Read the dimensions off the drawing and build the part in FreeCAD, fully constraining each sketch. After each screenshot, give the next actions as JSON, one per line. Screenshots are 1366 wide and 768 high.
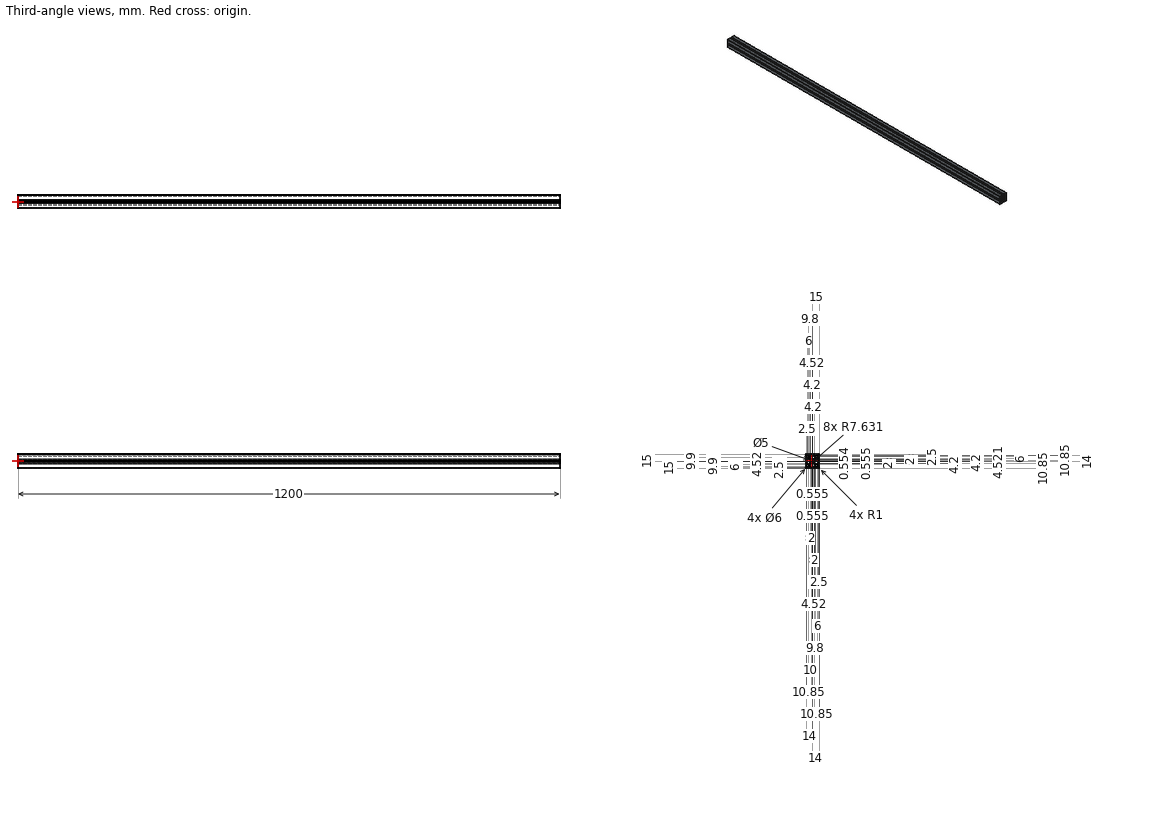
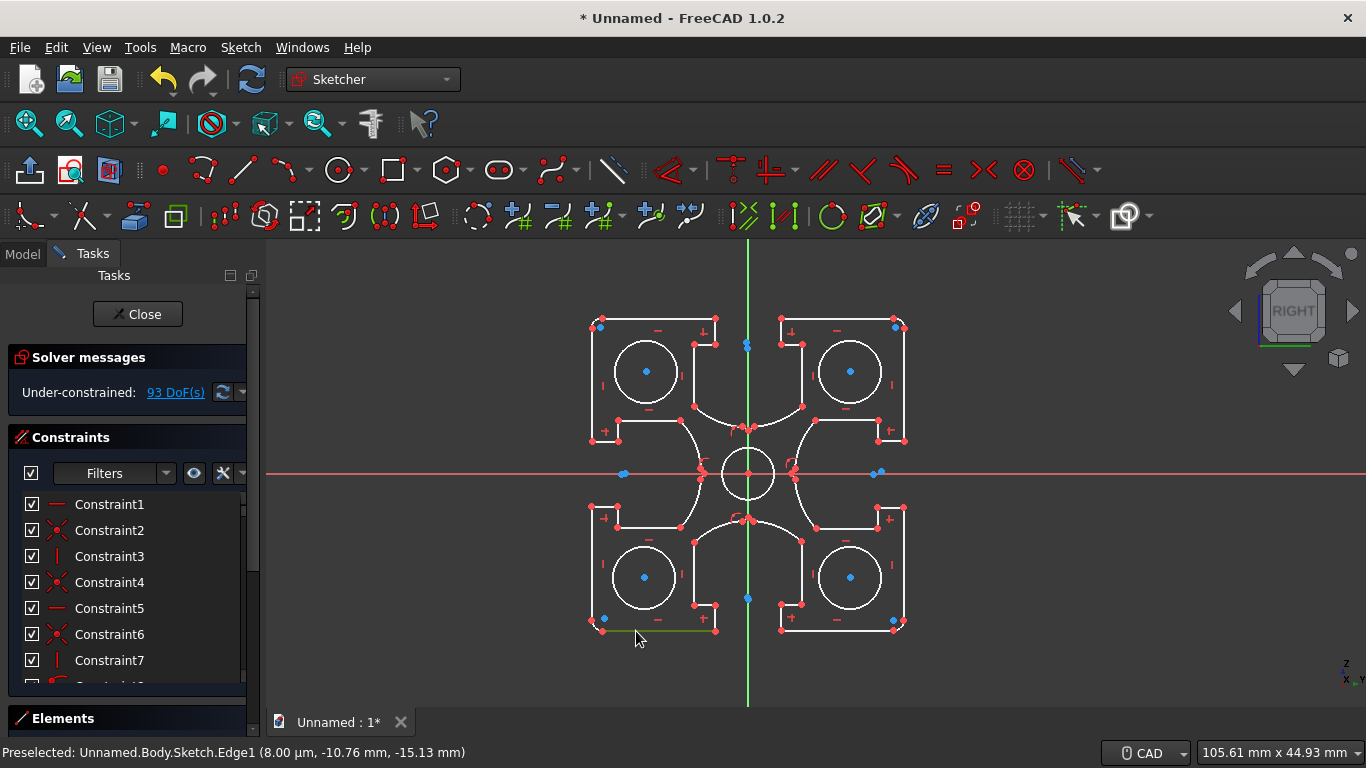
{"action": "scroll", "coordinate": [595, 628], "scroll_direction": "up", "scroll_amount": 3}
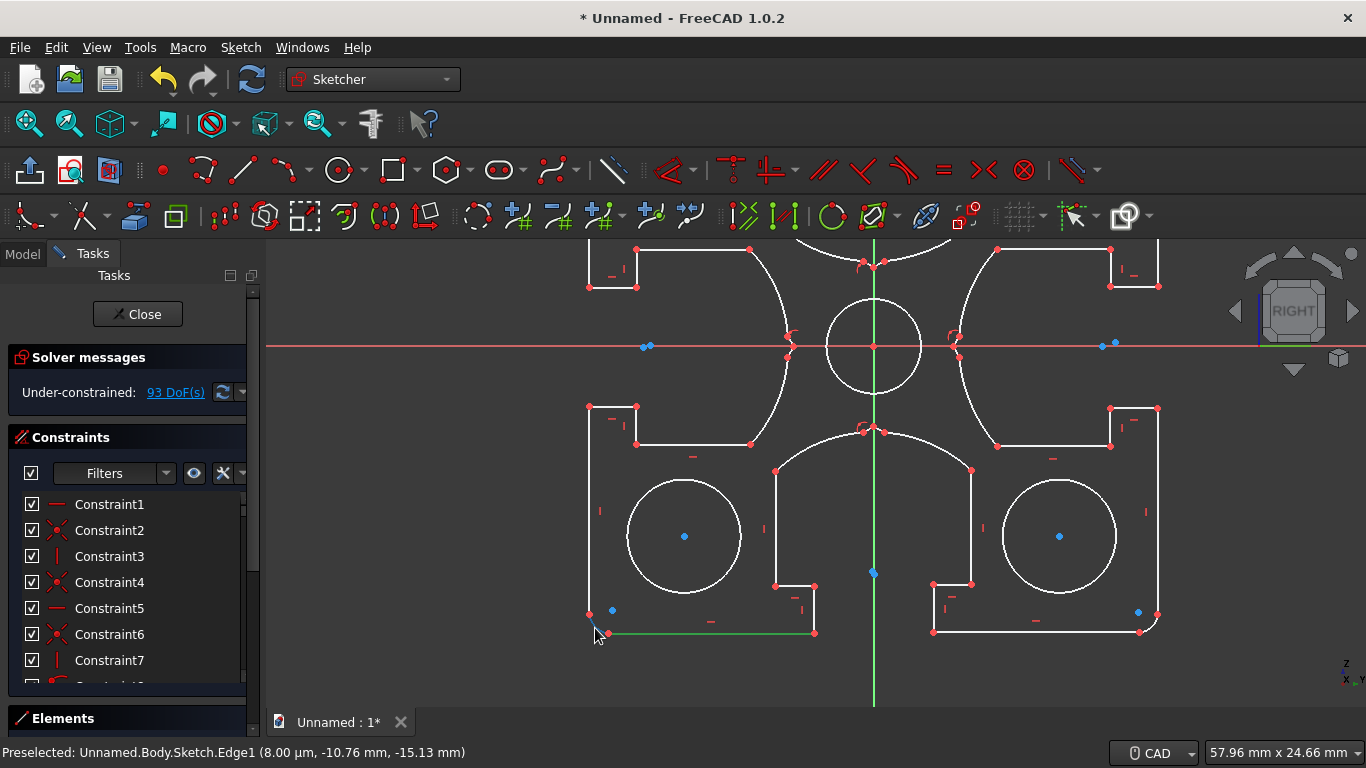
{"action": "left_click", "coordinate": [596, 627]}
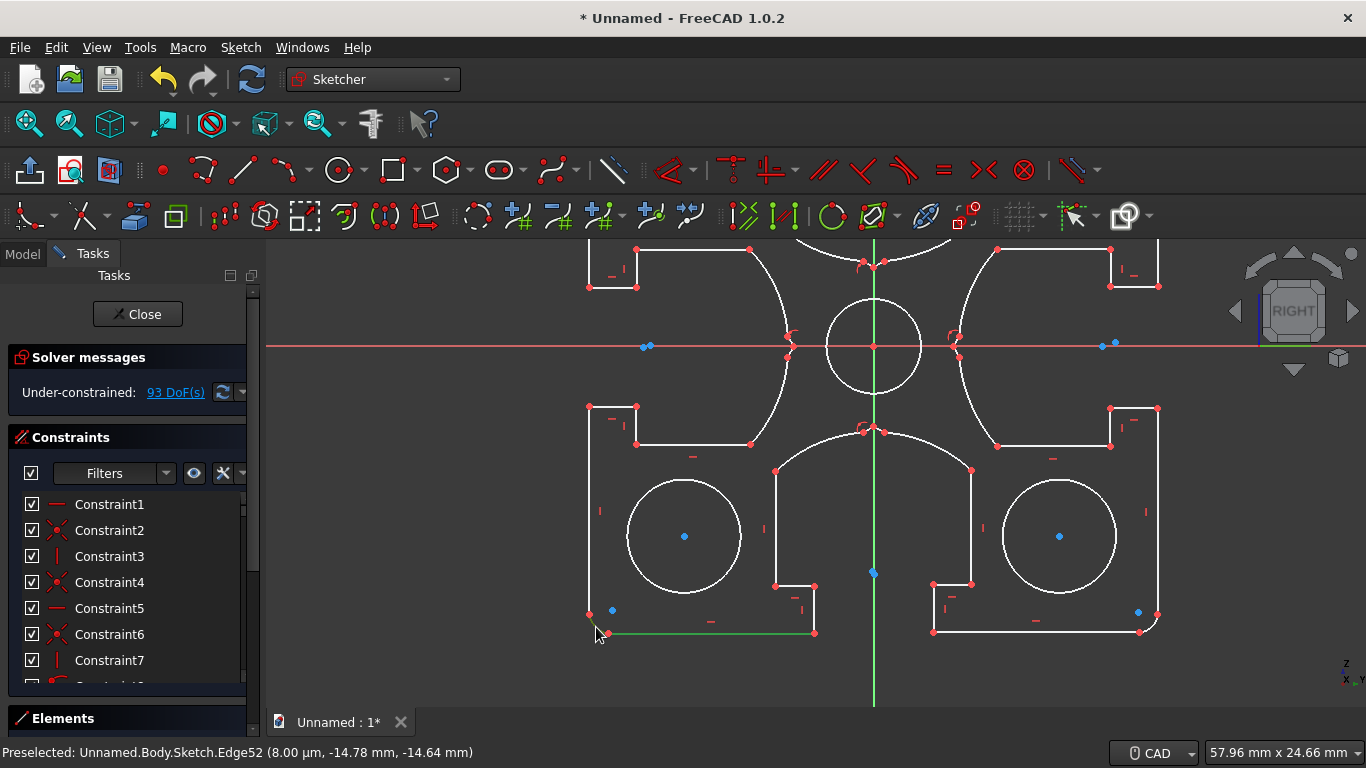
{"action": "left_click", "coordinate": [904, 170]}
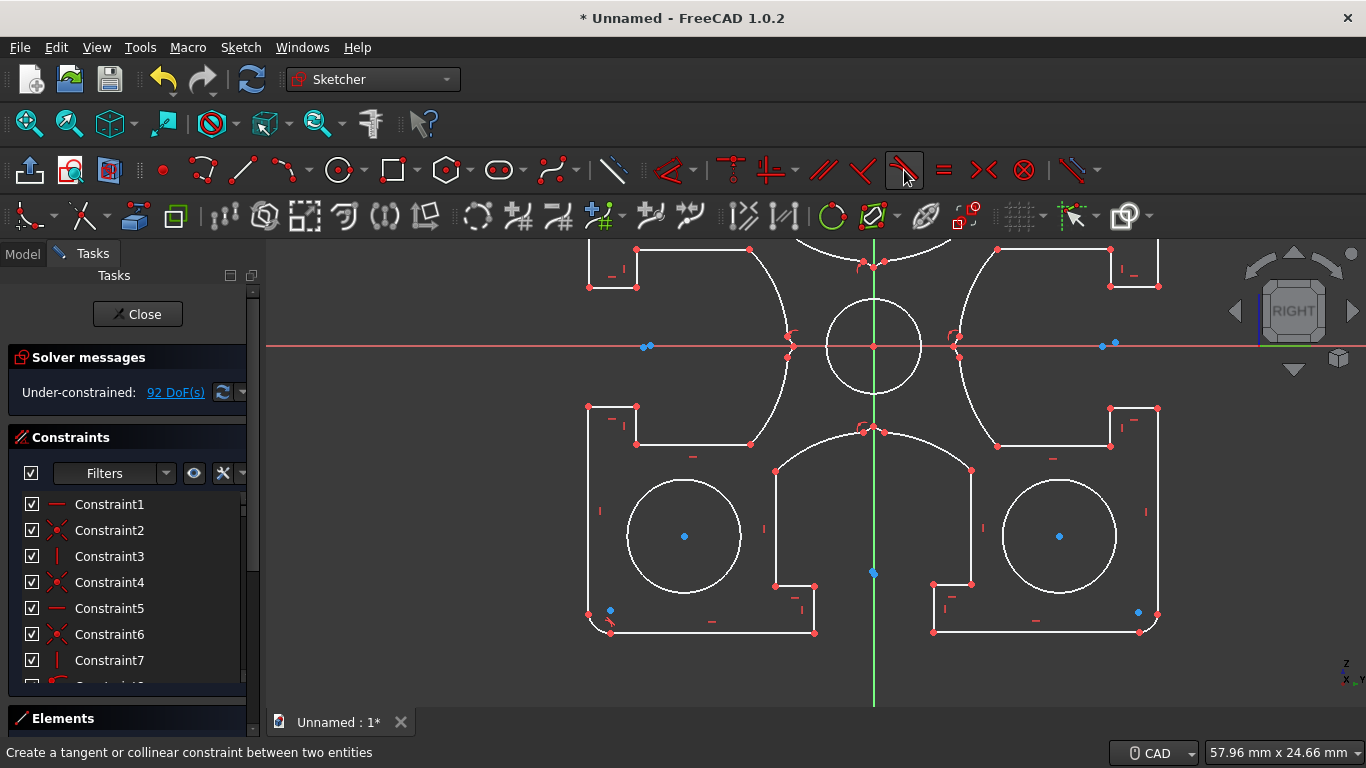
{"action": "left_click", "coordinate": [995, 632]}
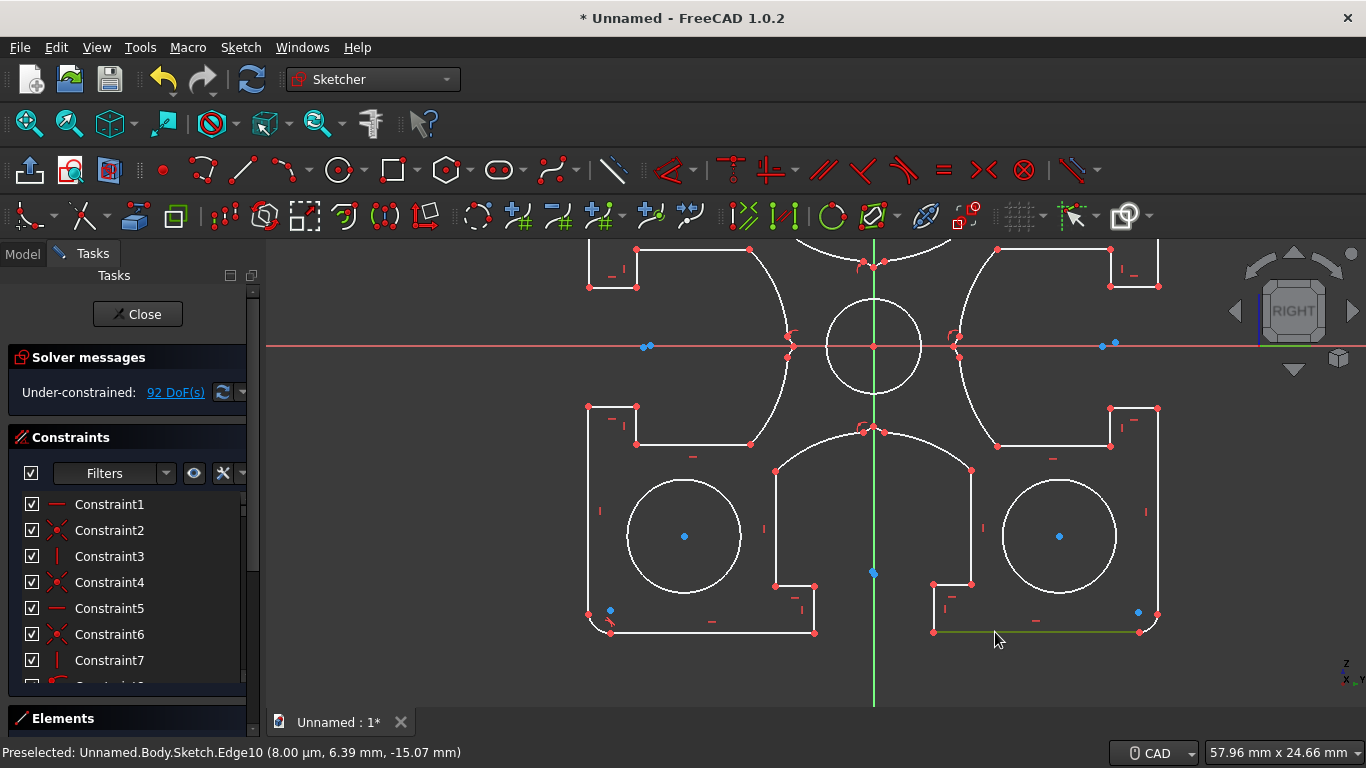
{"action": "left_click", "coordinate": [1152, 627]}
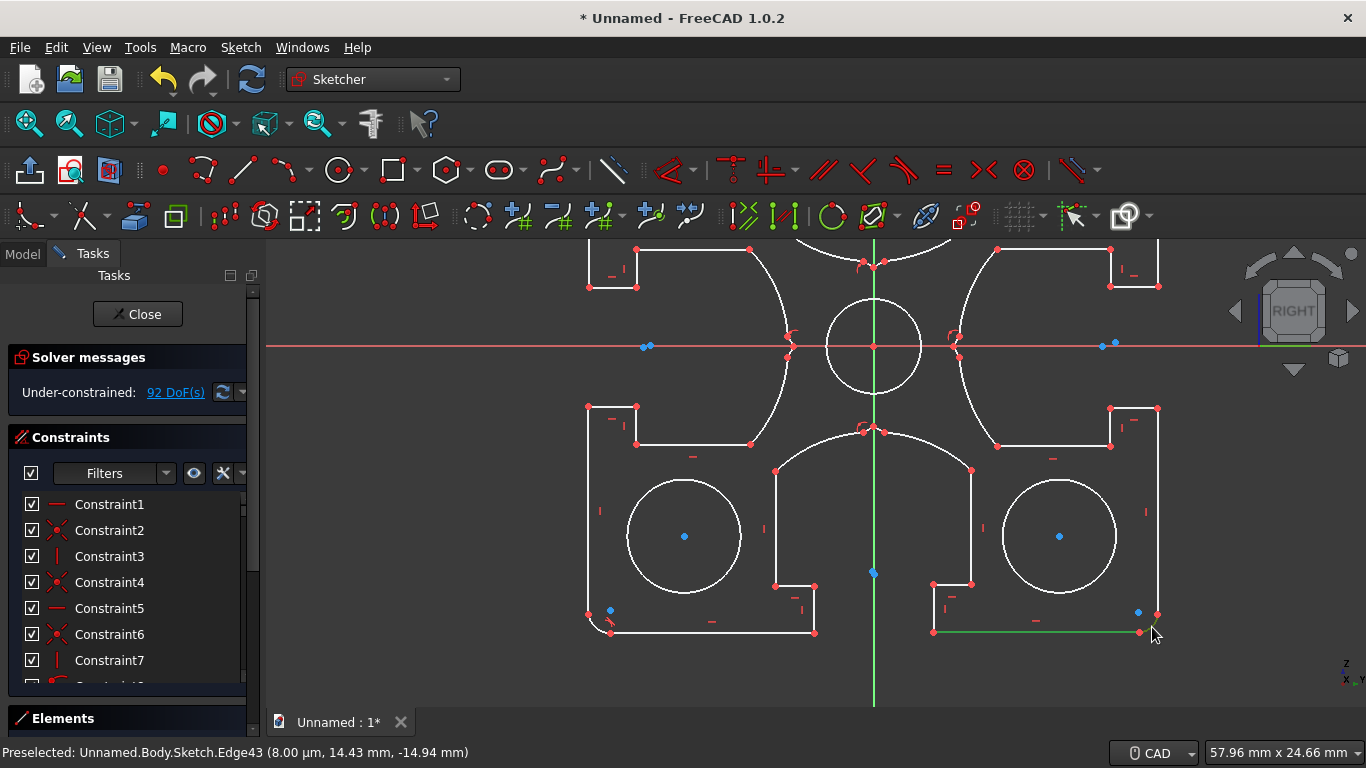
{"action": "left_click", "coordinate": [904, 170]}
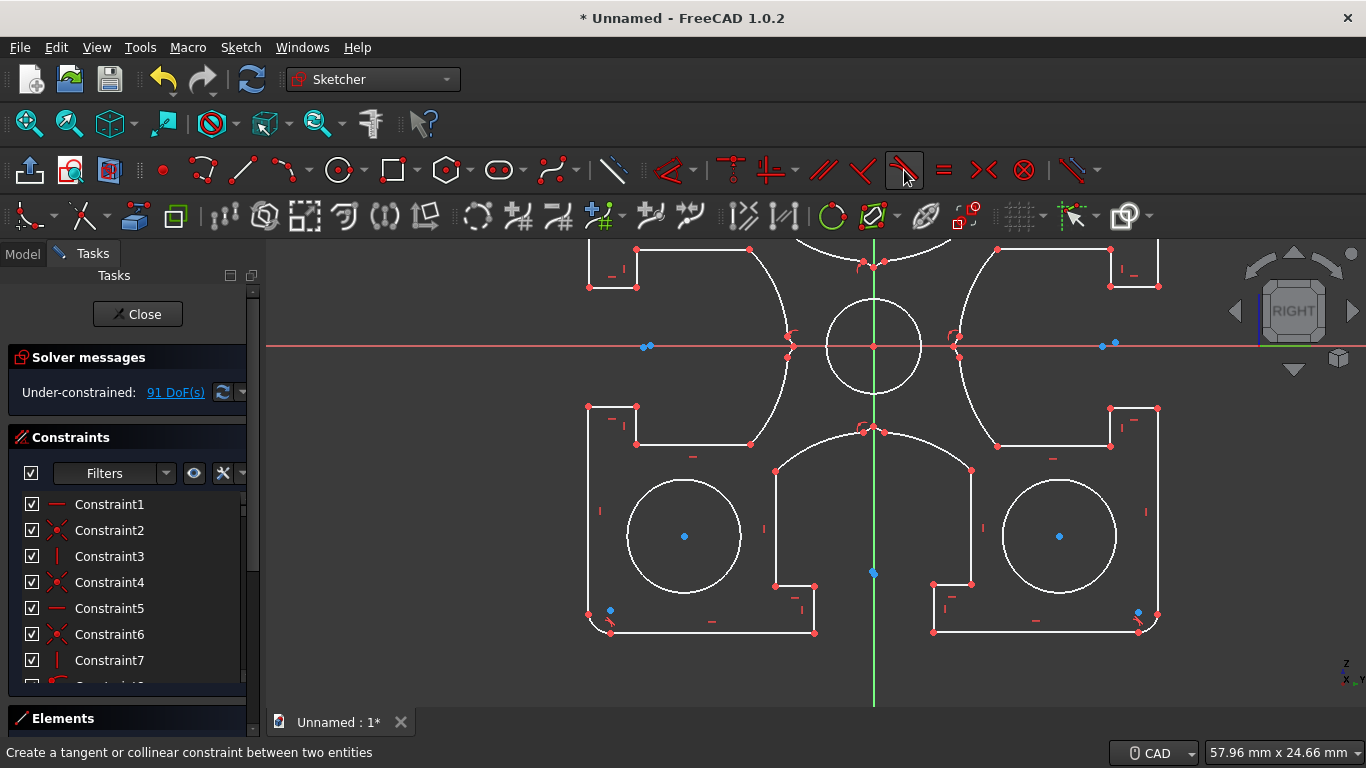
{"action": "left_click", "coordinate": [1158, 552]}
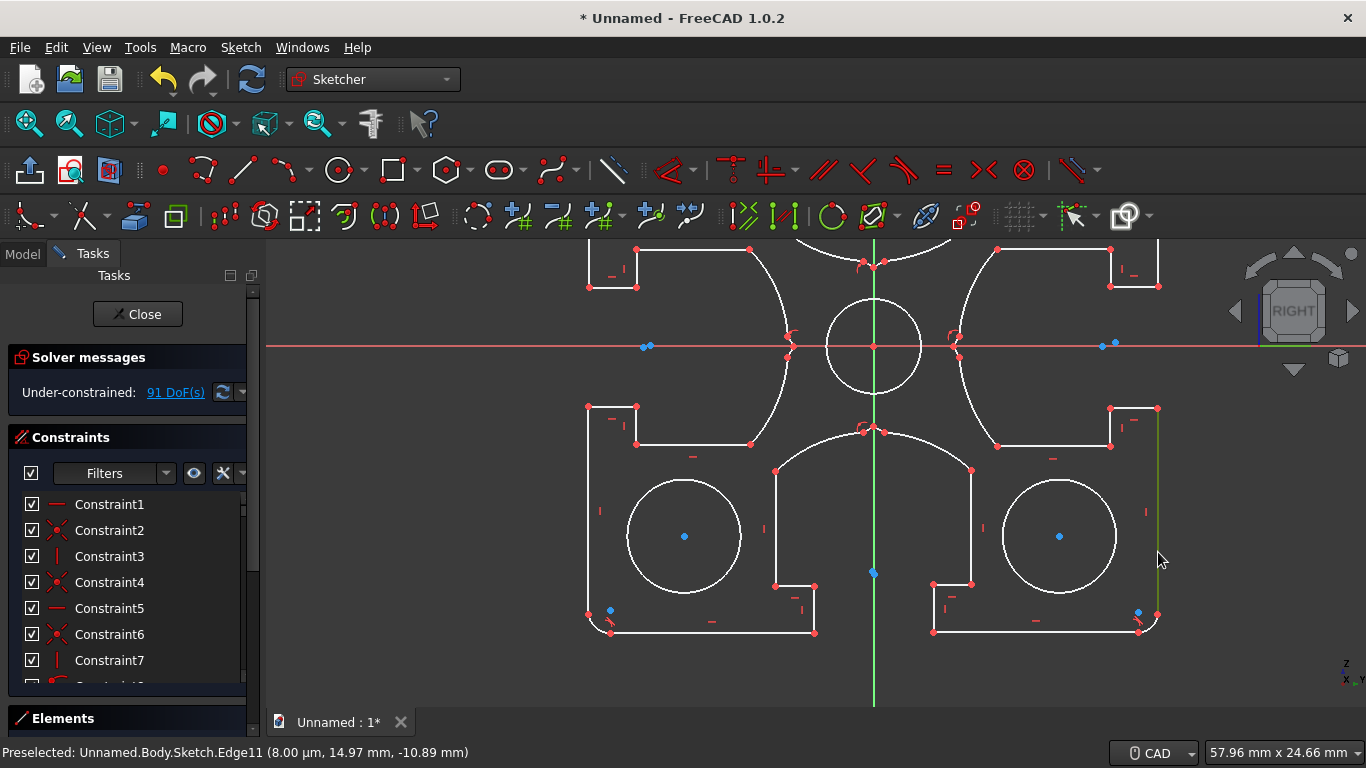
{"action": "left_click", "coordinate": [1152, 627]}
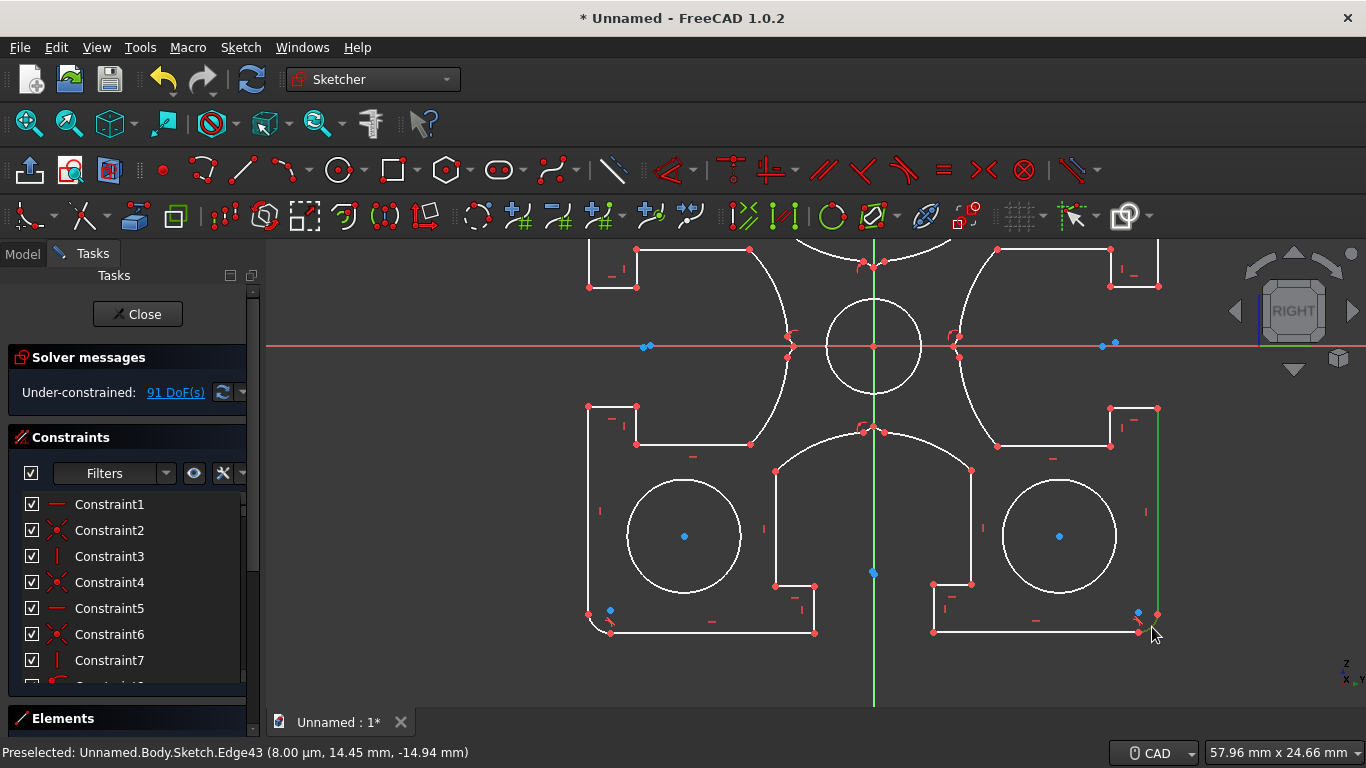
{"action": "left_click", "coordinate": [904, 170]}